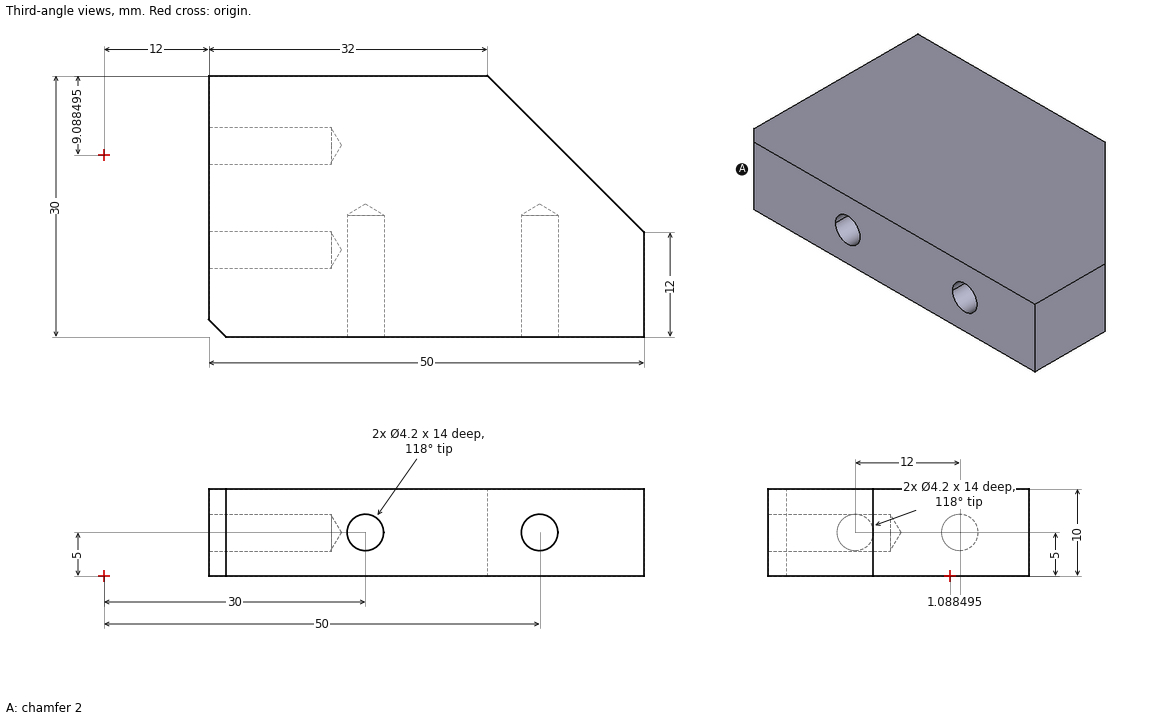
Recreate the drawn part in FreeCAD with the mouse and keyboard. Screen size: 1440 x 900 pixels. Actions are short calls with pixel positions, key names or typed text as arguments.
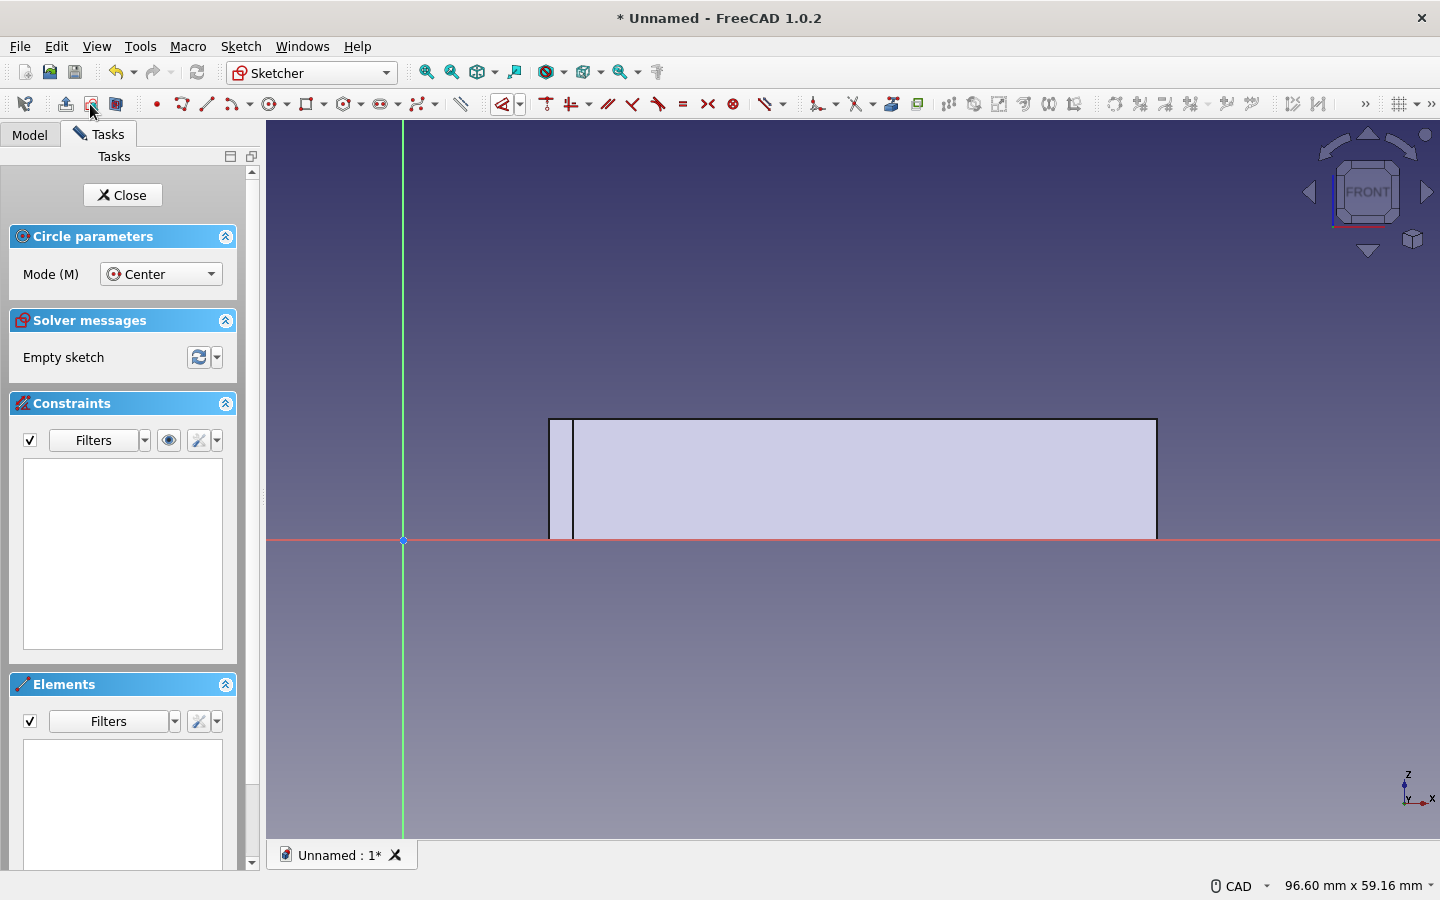
click(768, 480)
move(786, 461)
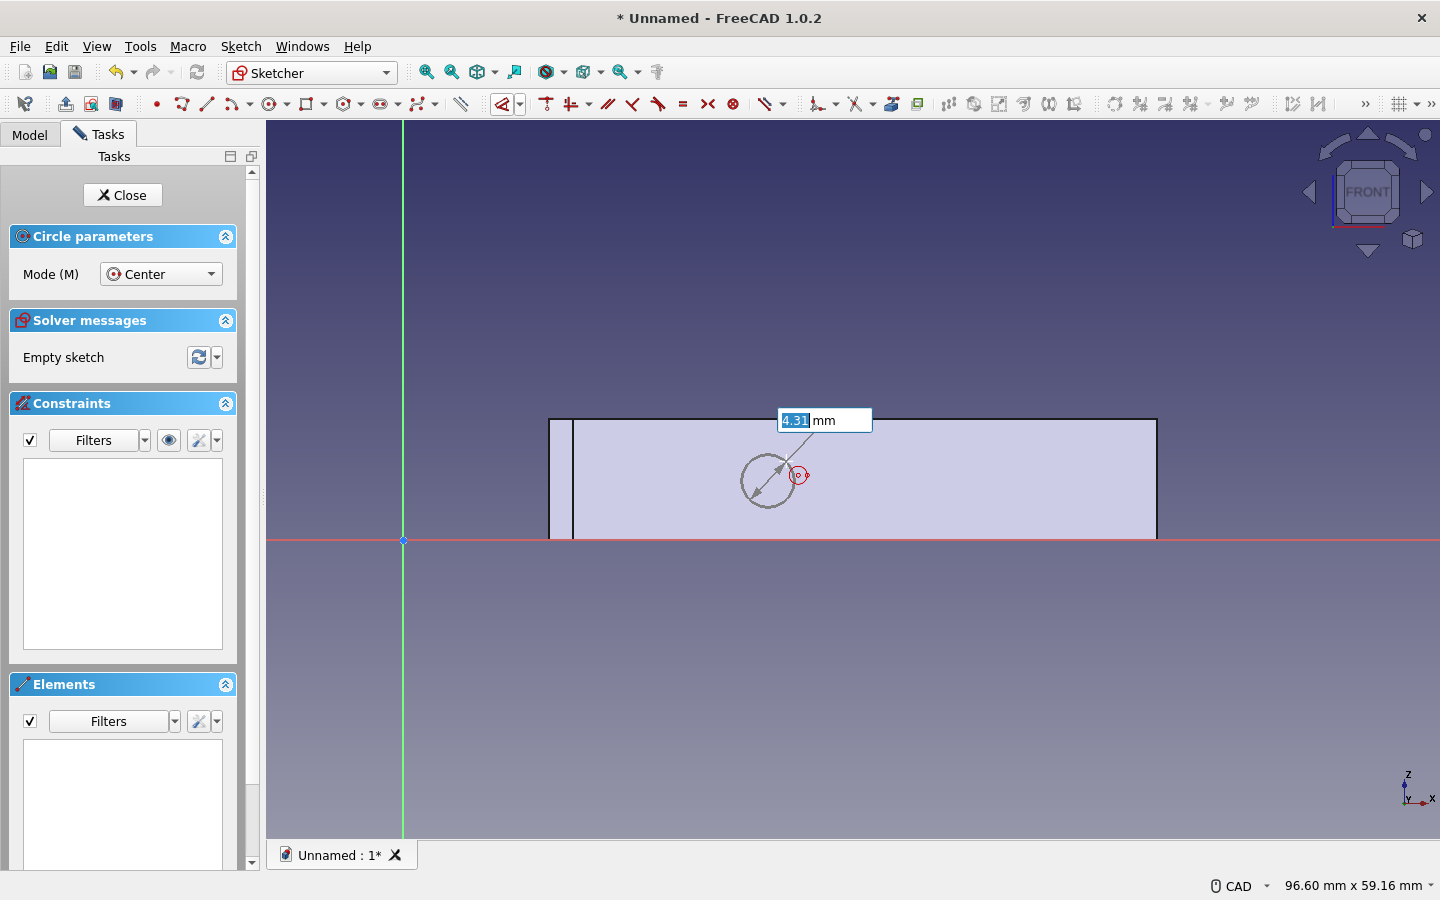
text(4.2)
key(Return)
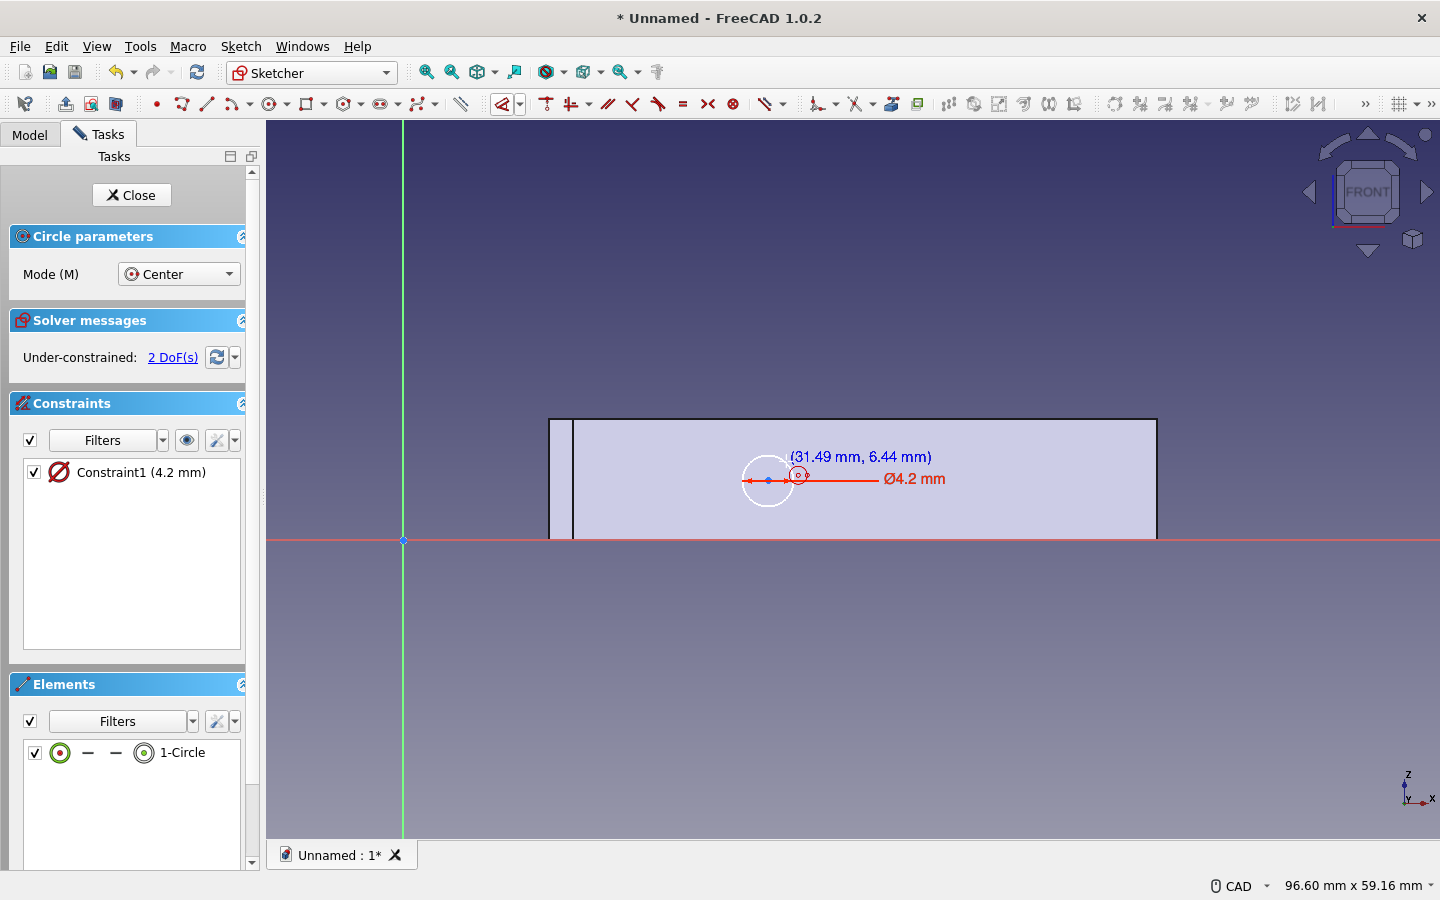
click(1011, 480)
move(1029, 461)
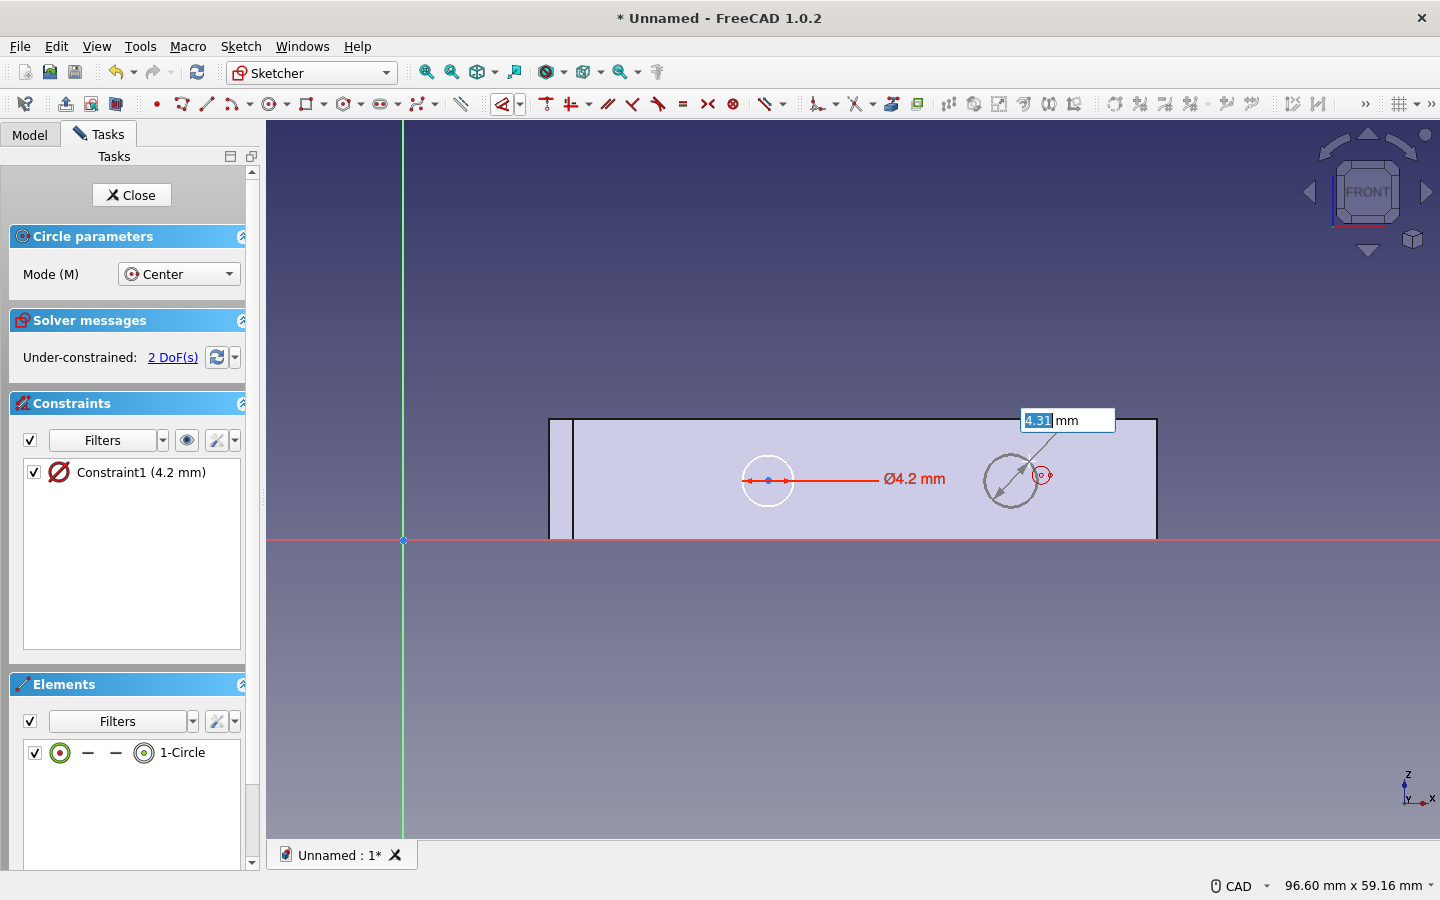
text(4.2)
key(Return)
key(Escape)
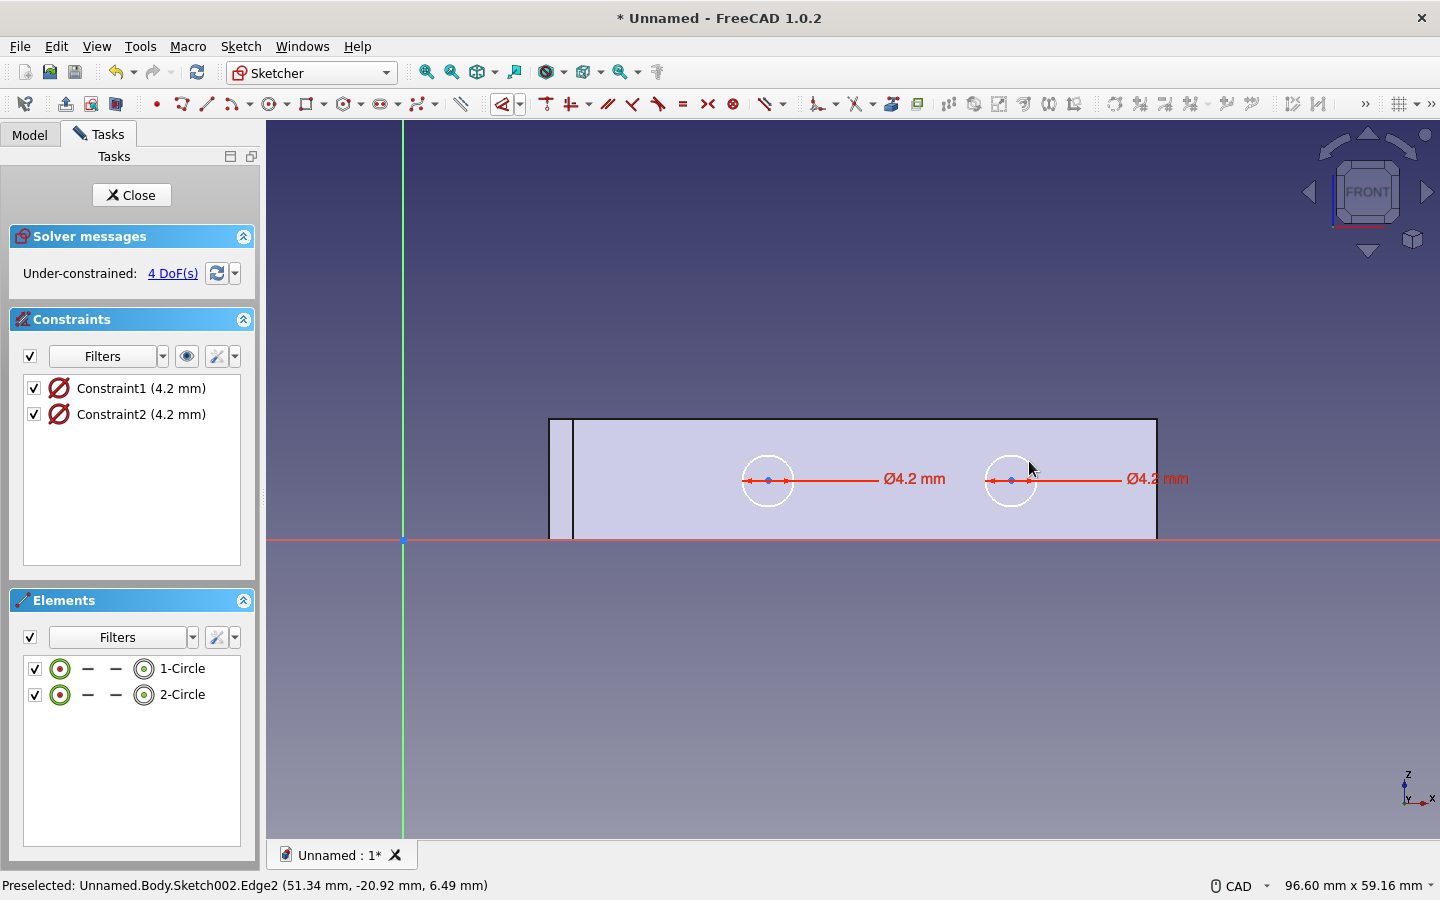
click(768, 481)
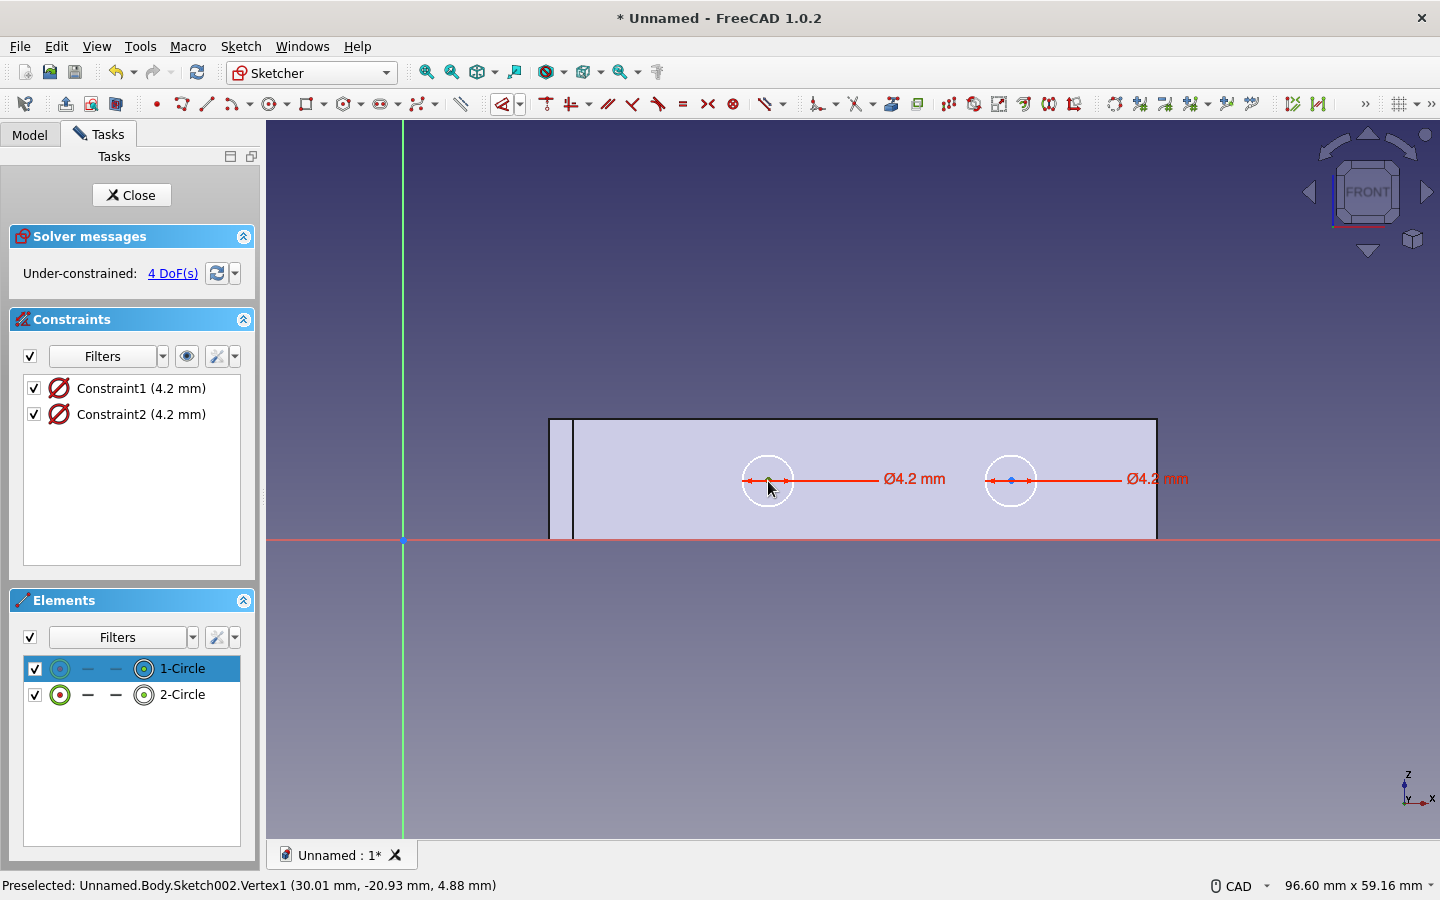
click(1011, 481)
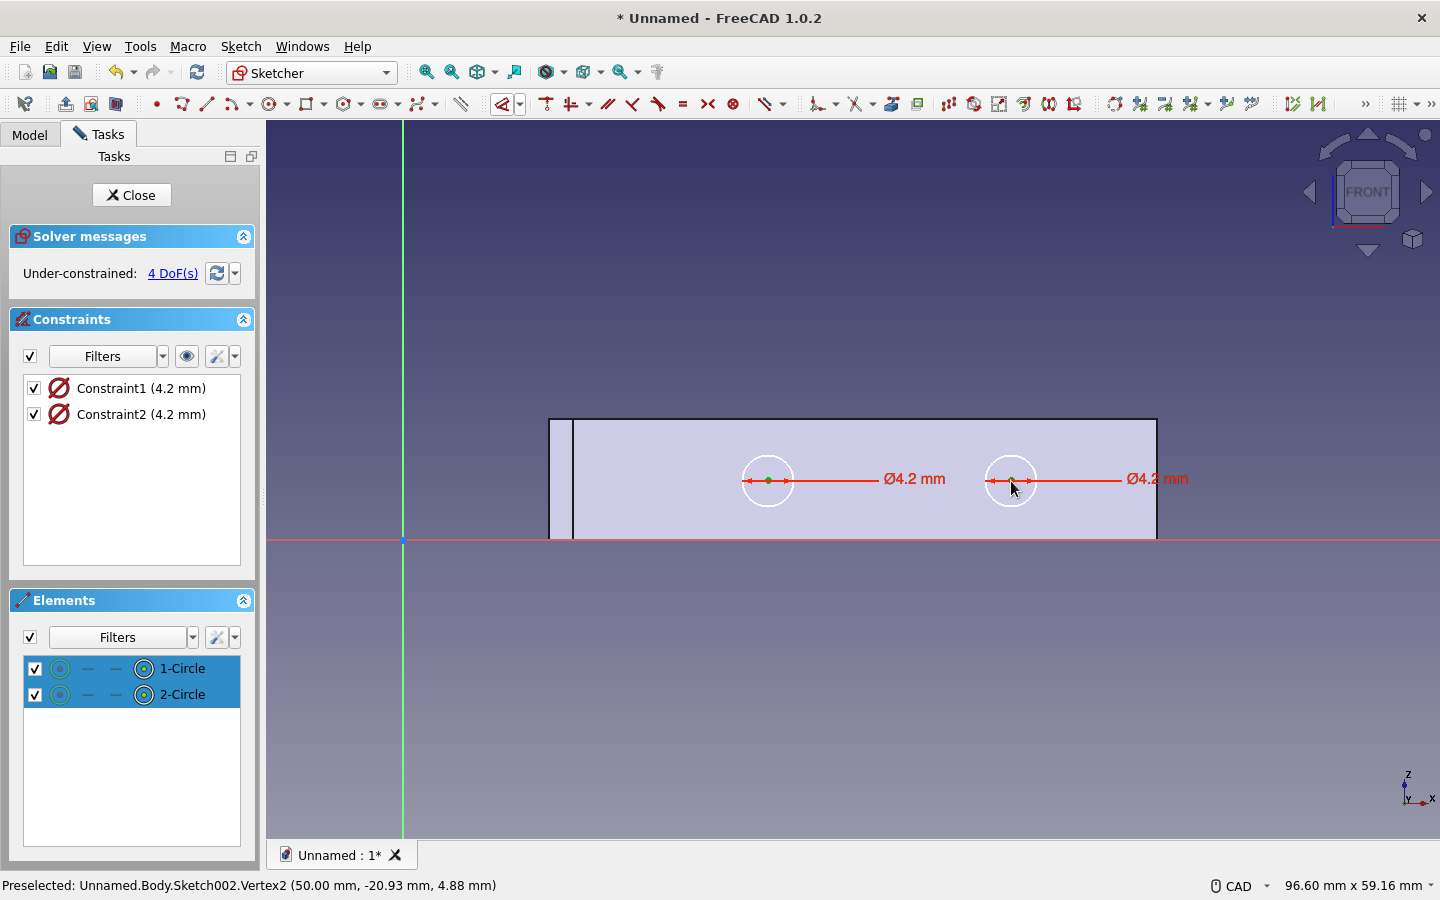
key(h)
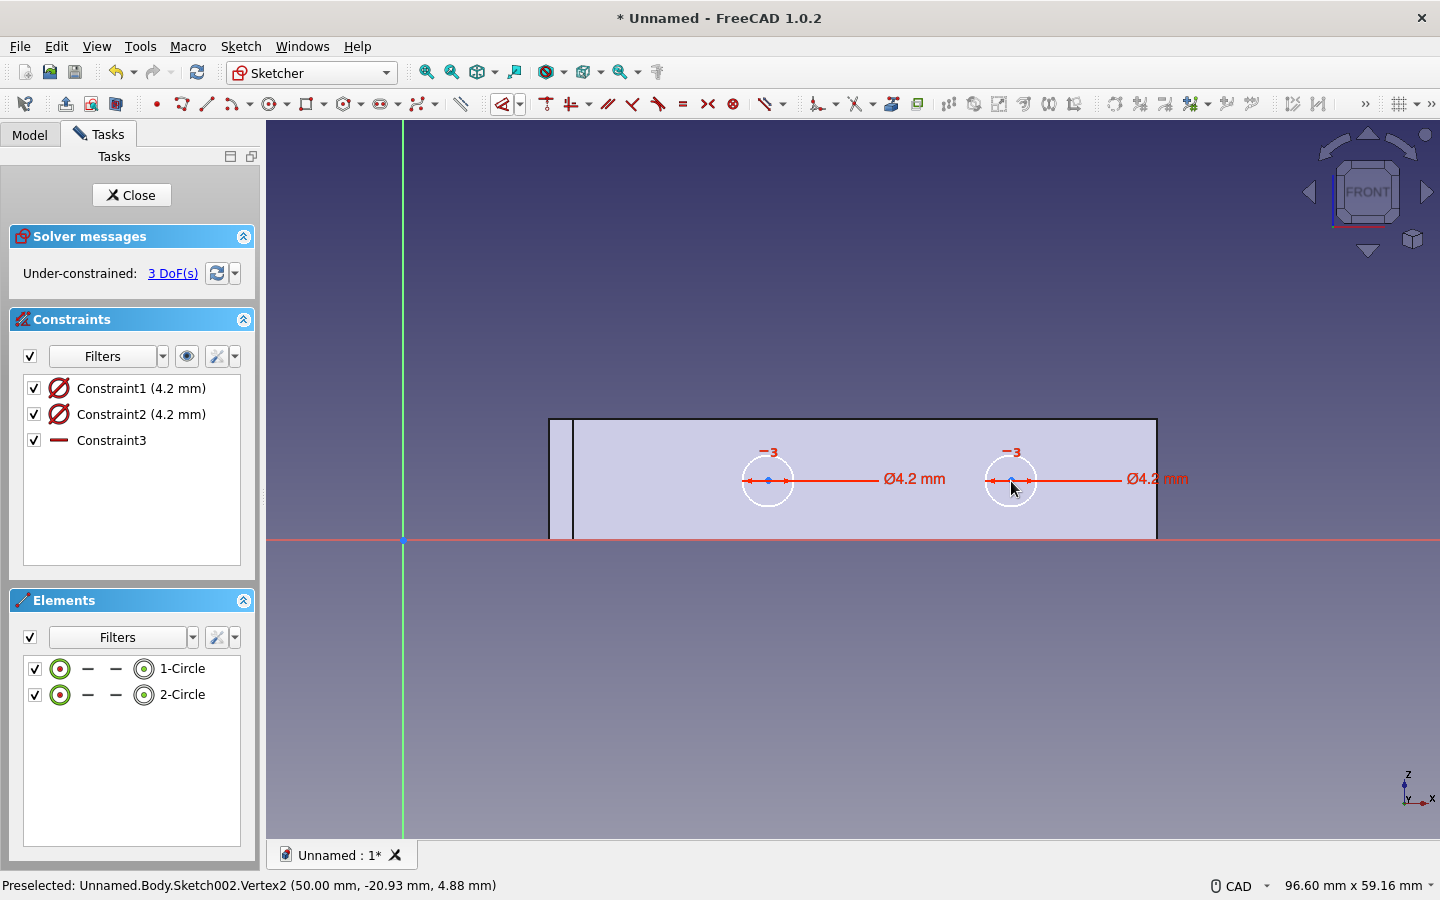
click(768, 481)